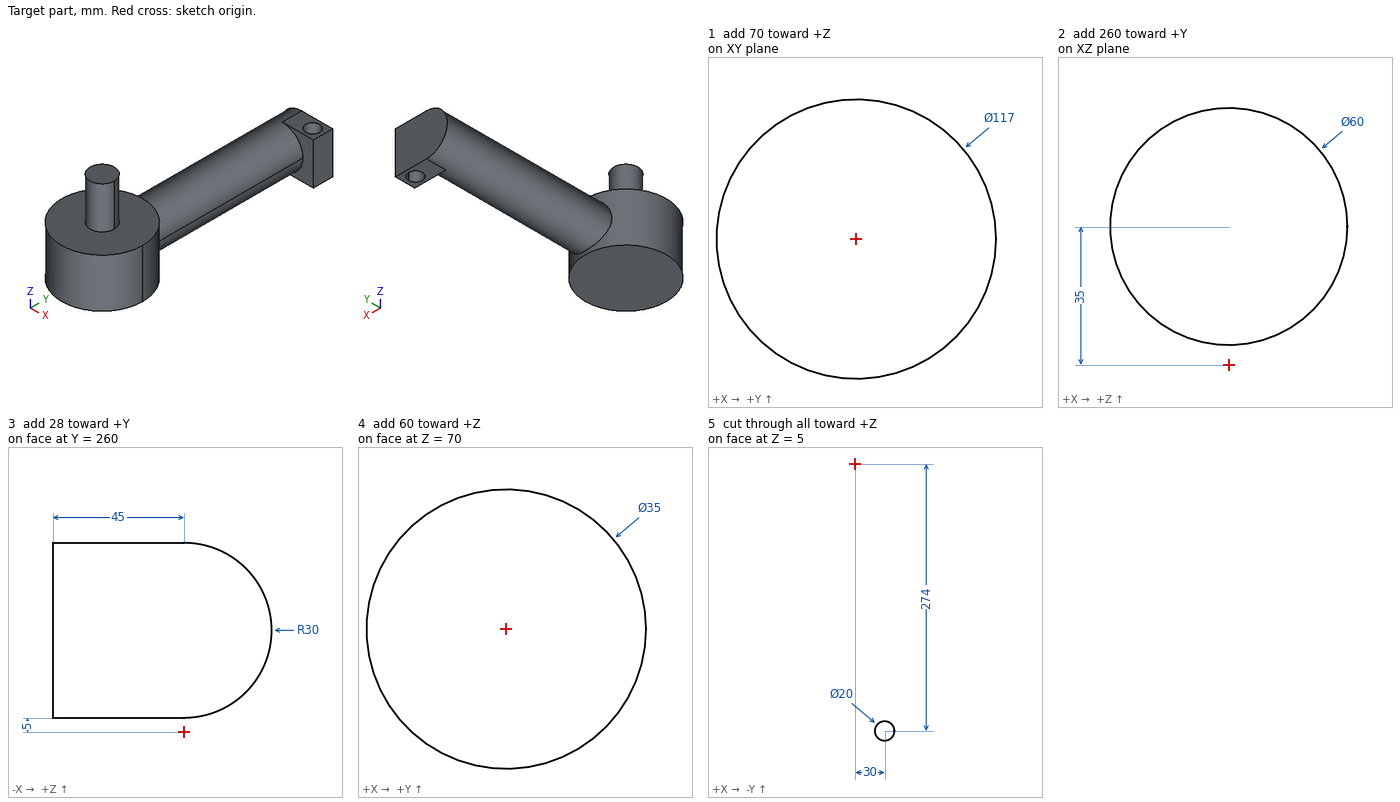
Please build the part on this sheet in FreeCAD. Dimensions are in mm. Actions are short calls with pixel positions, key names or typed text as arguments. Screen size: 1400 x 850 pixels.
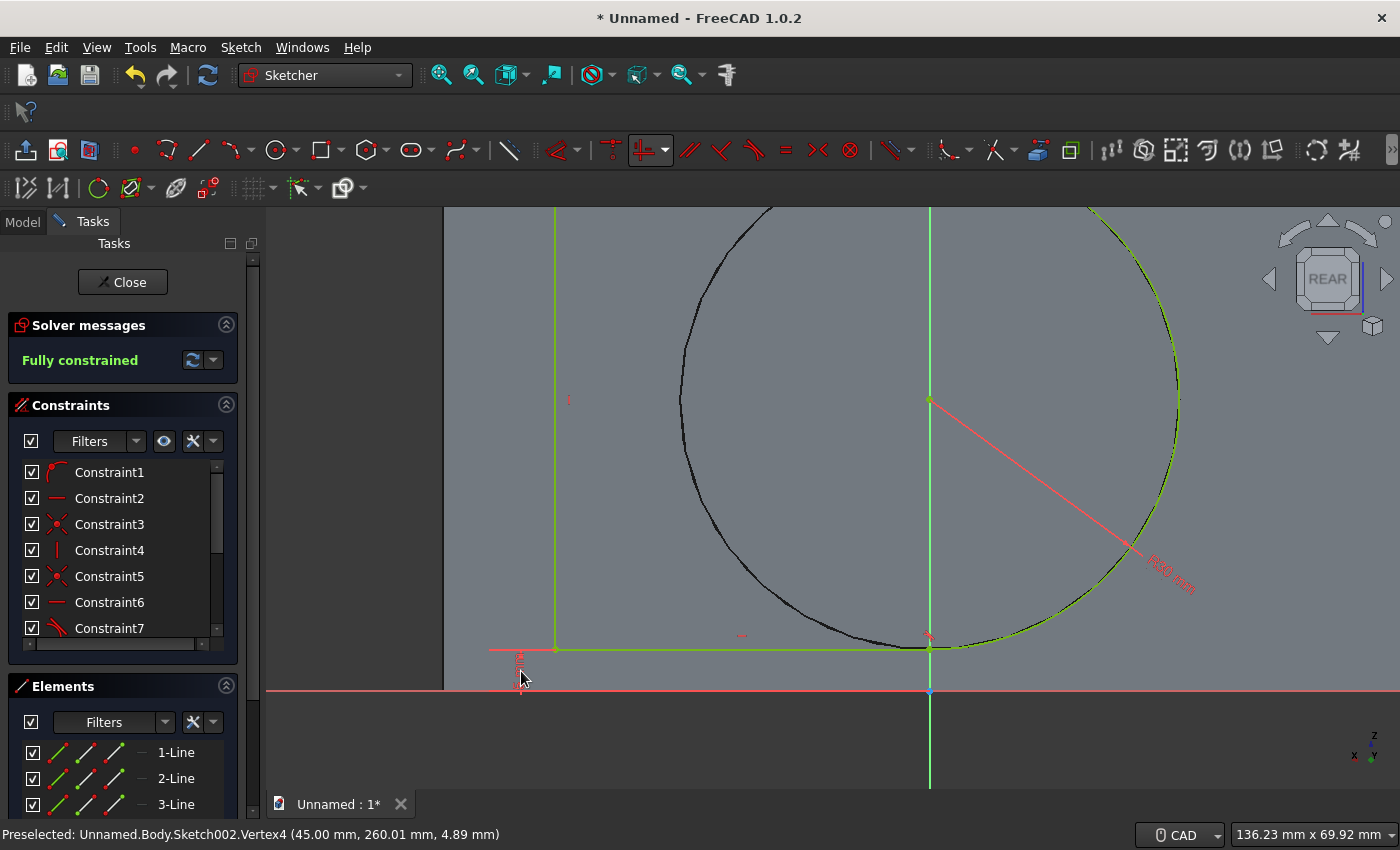
click(123, 282)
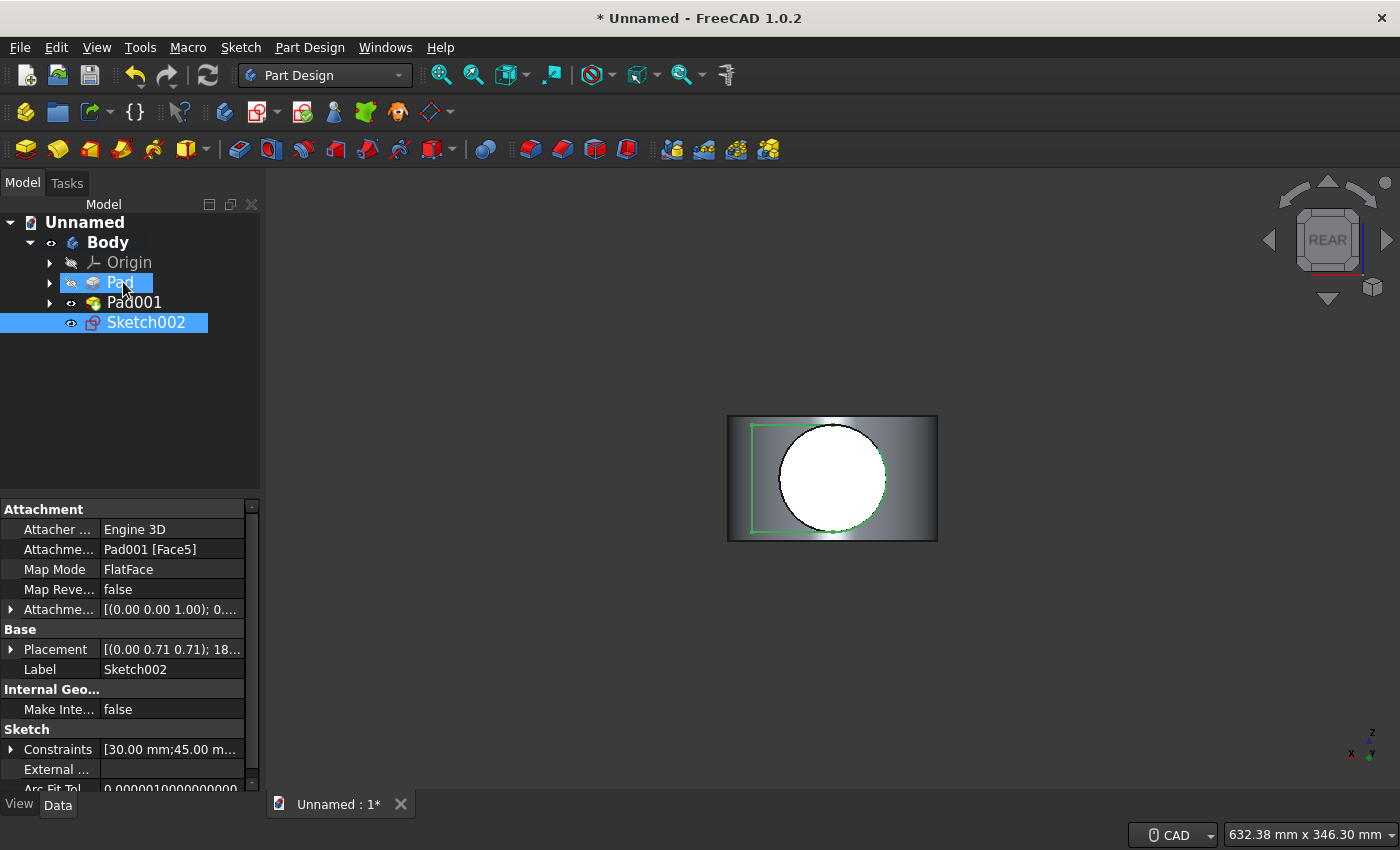
click(26, 150)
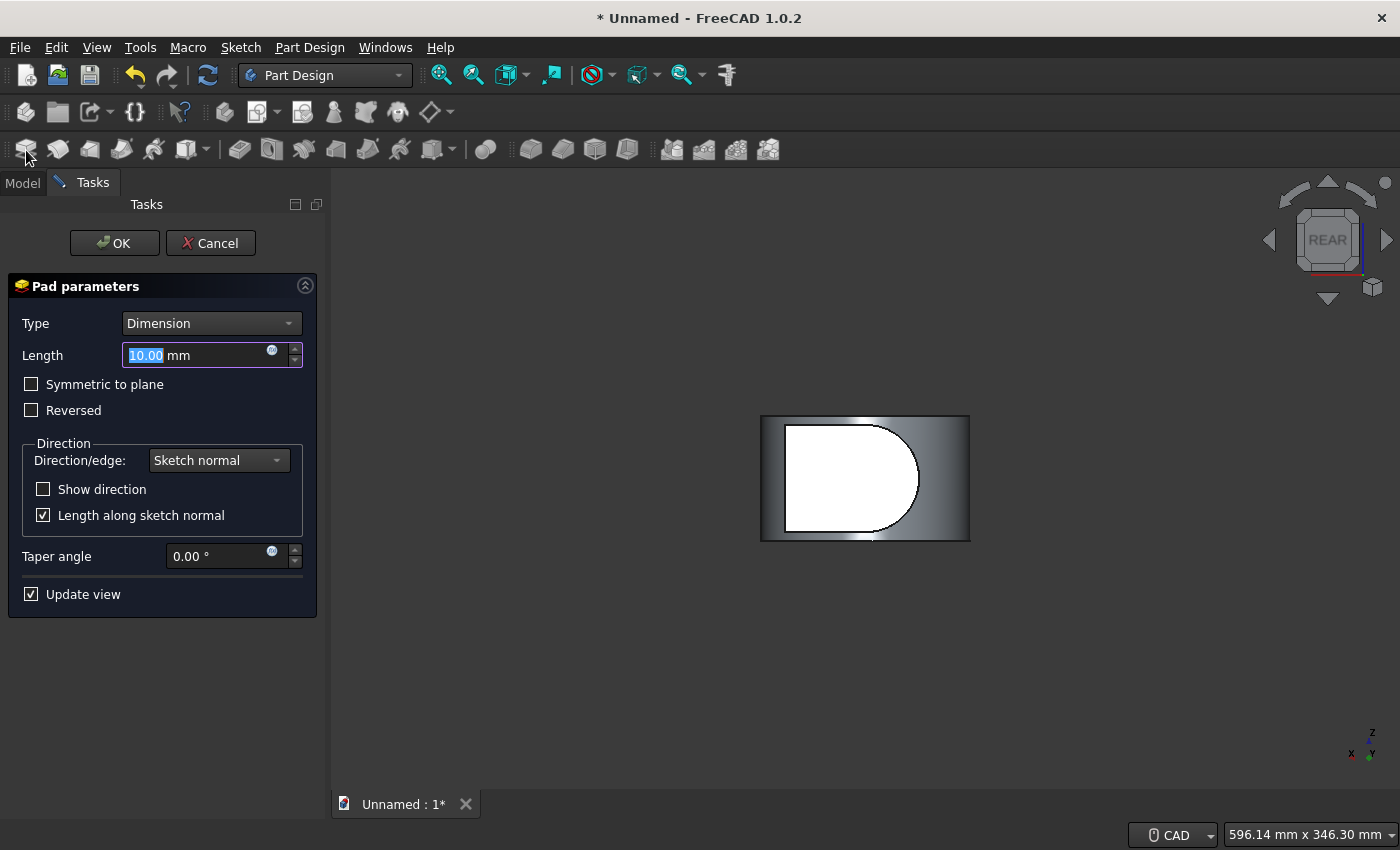
text(28)
key(Tab)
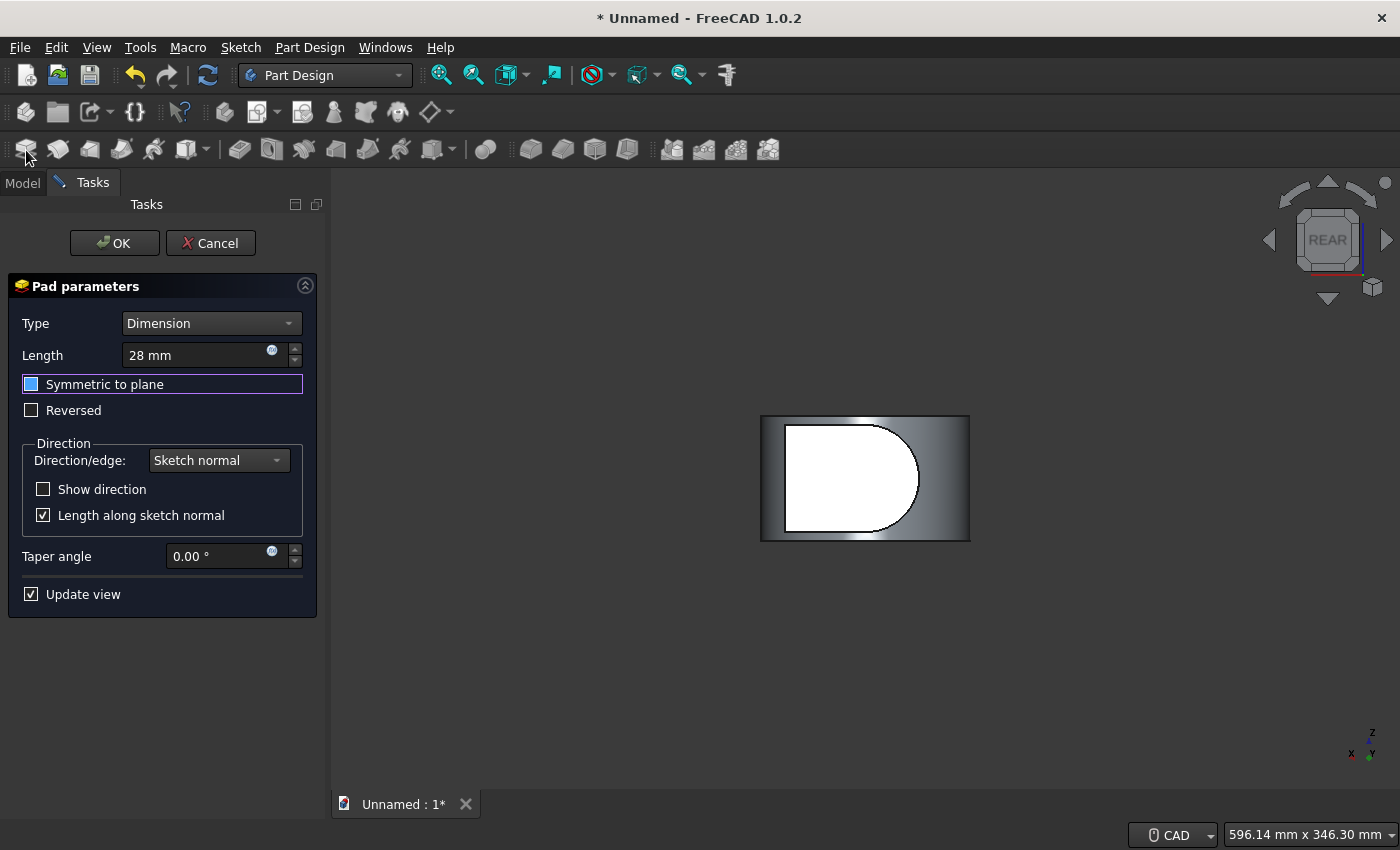
click(115, 243)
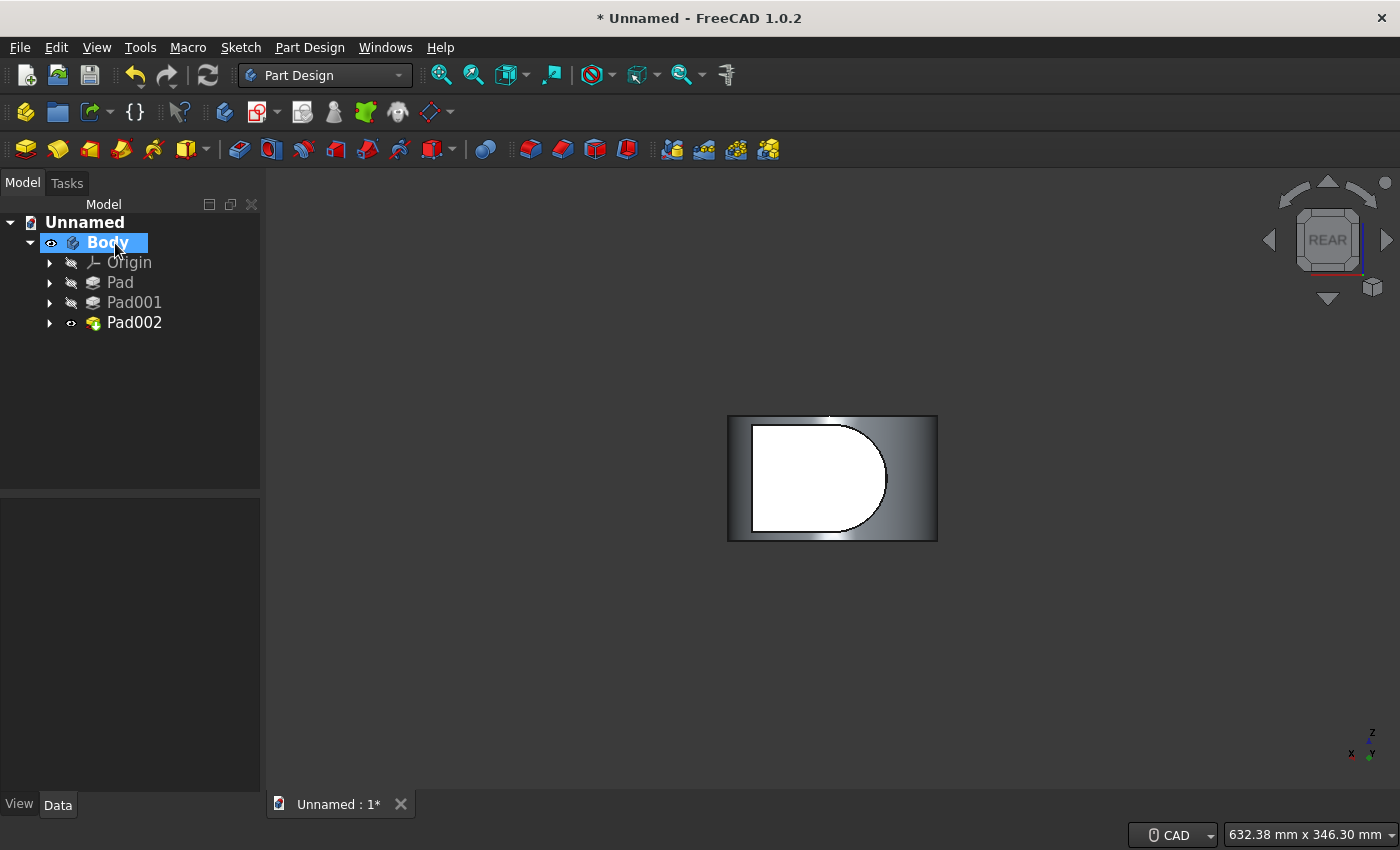
click(442, 76)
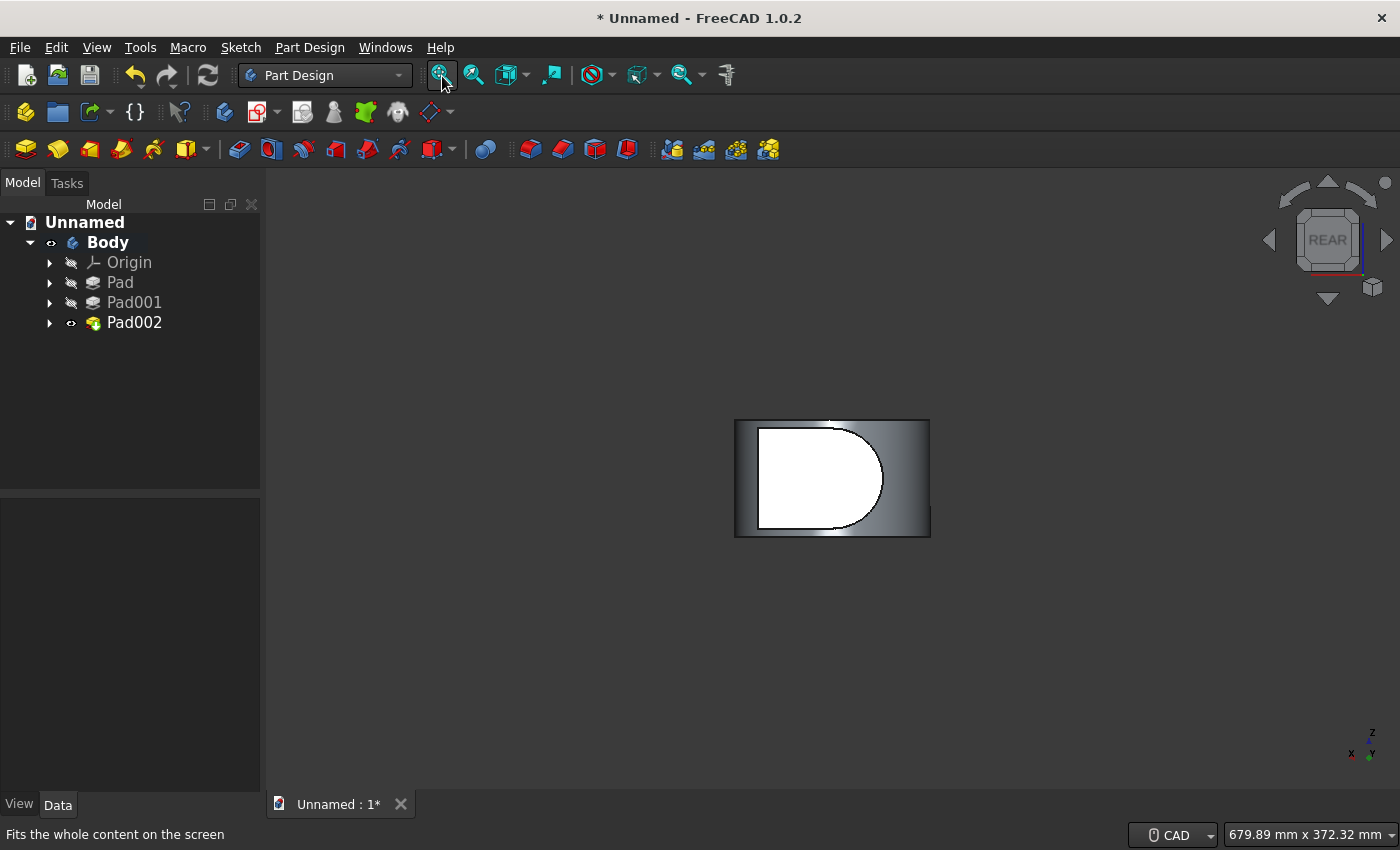
key(0)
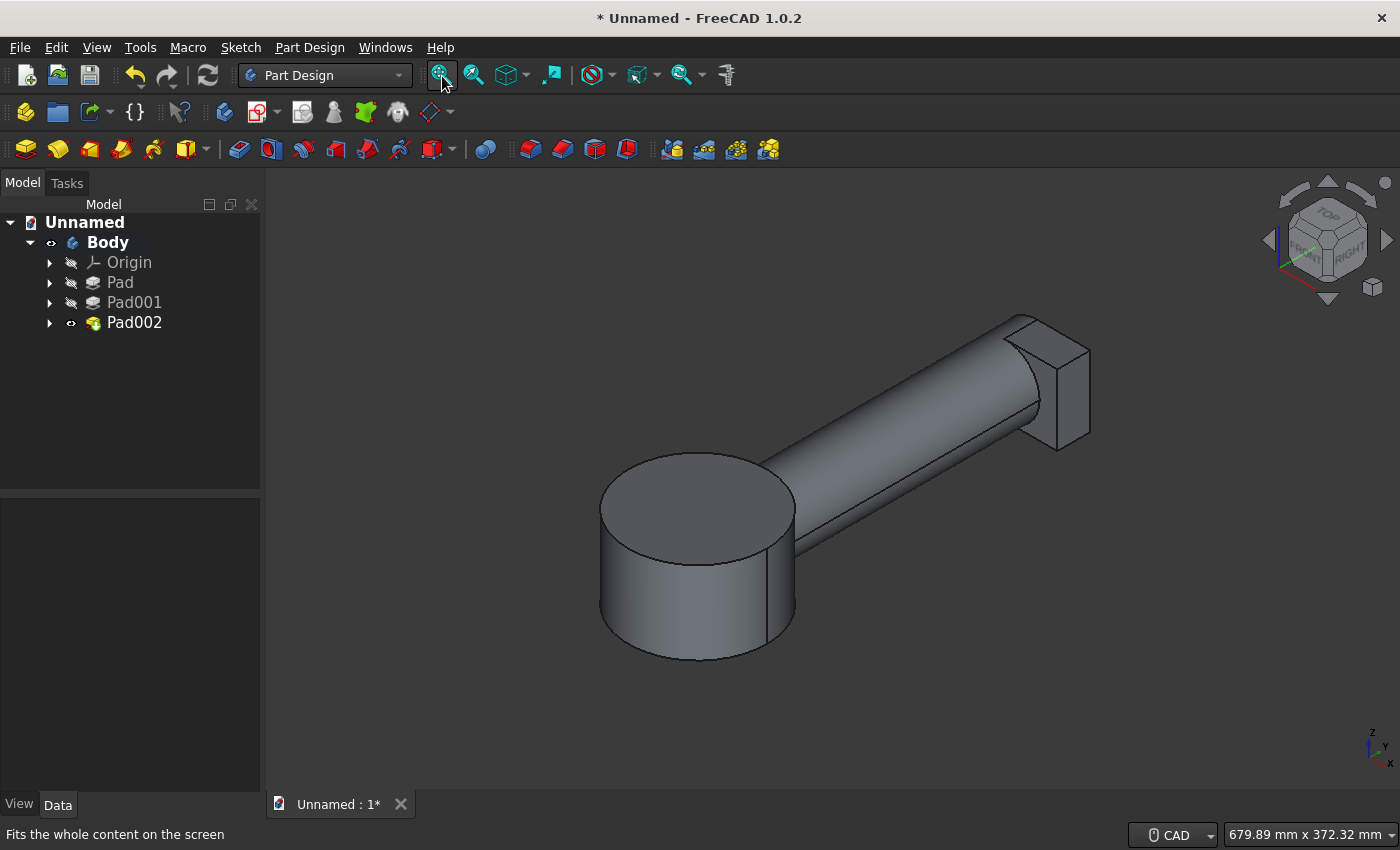
click(698, 508)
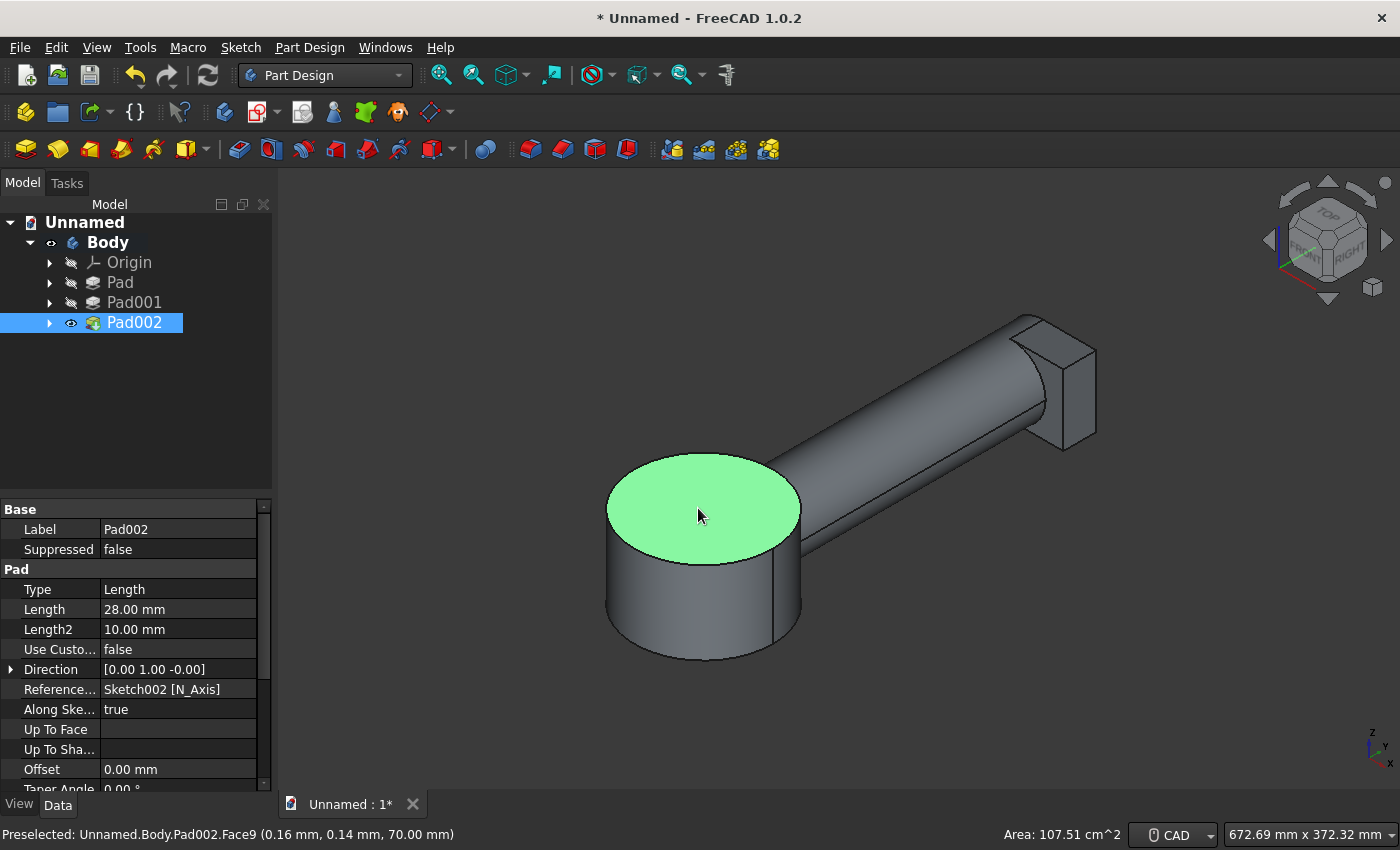
click(258, 112)